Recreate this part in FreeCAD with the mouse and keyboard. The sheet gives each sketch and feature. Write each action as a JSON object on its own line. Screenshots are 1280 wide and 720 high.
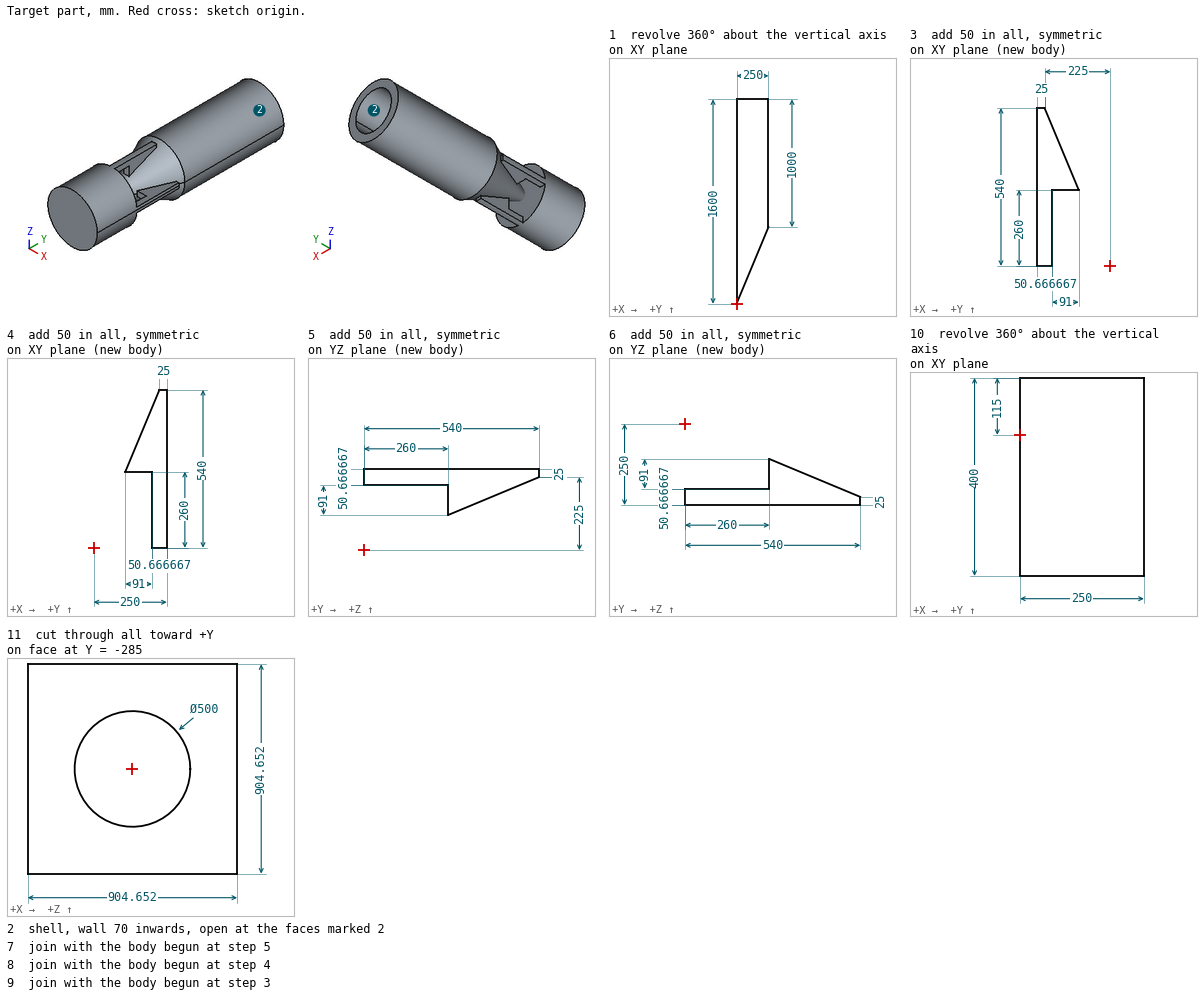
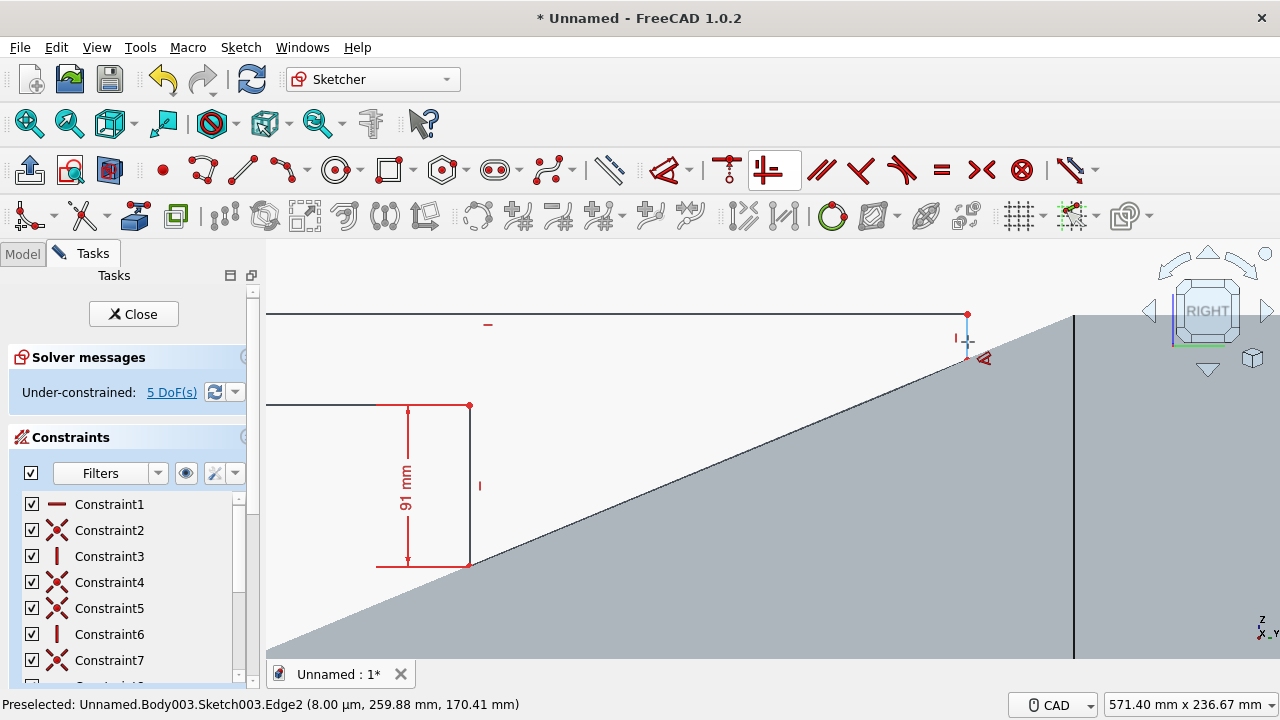
{"action": "left_click", "coordinate": [967, 342]}
{"action": "left_click", "coordinate": [1001, 337]}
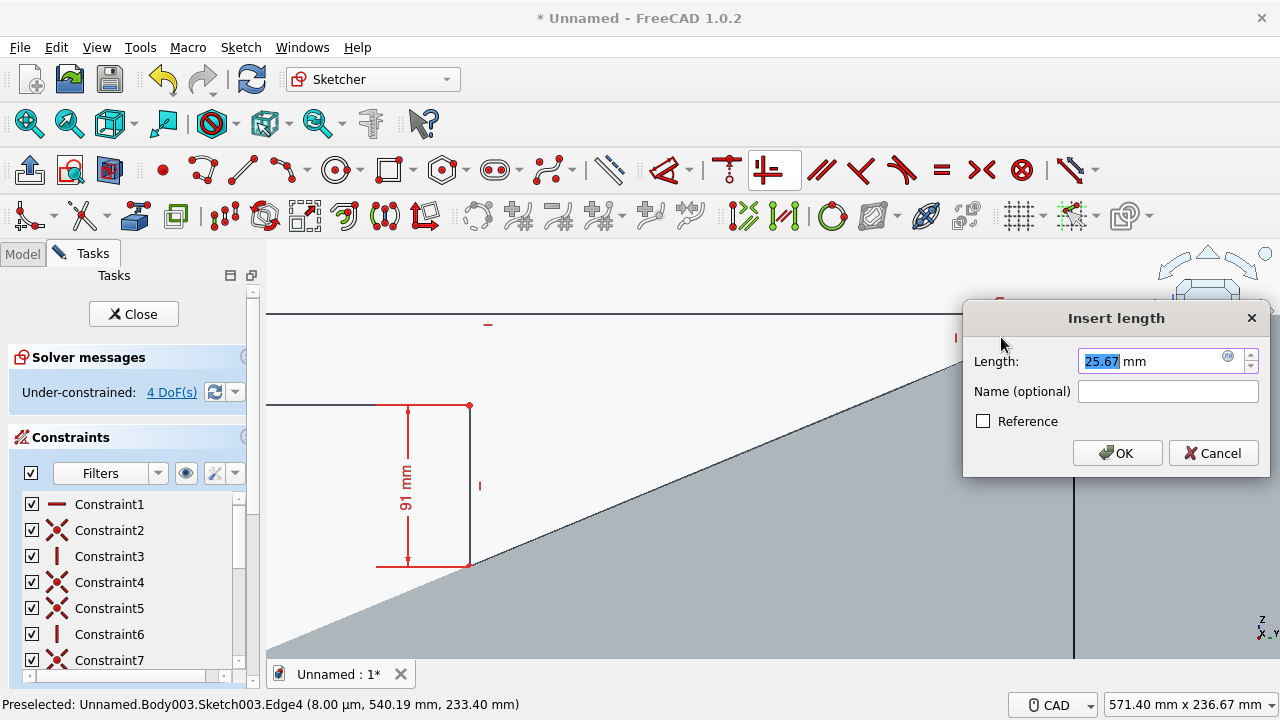
{"action": "type", "text": "25"}
{"action": "key", "text": "Return"}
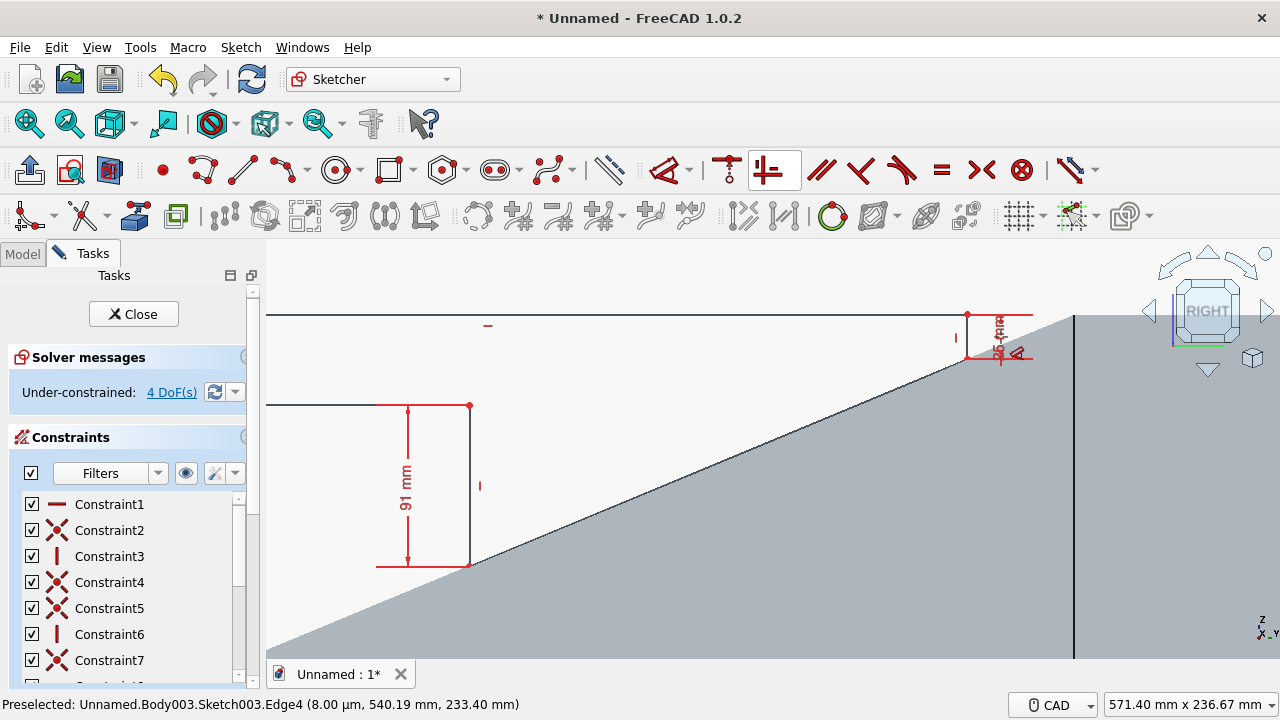
{"action": "left_click", "coordinate": [332, 405]}
{"action": "left_click", "coordinate": [382, 371]}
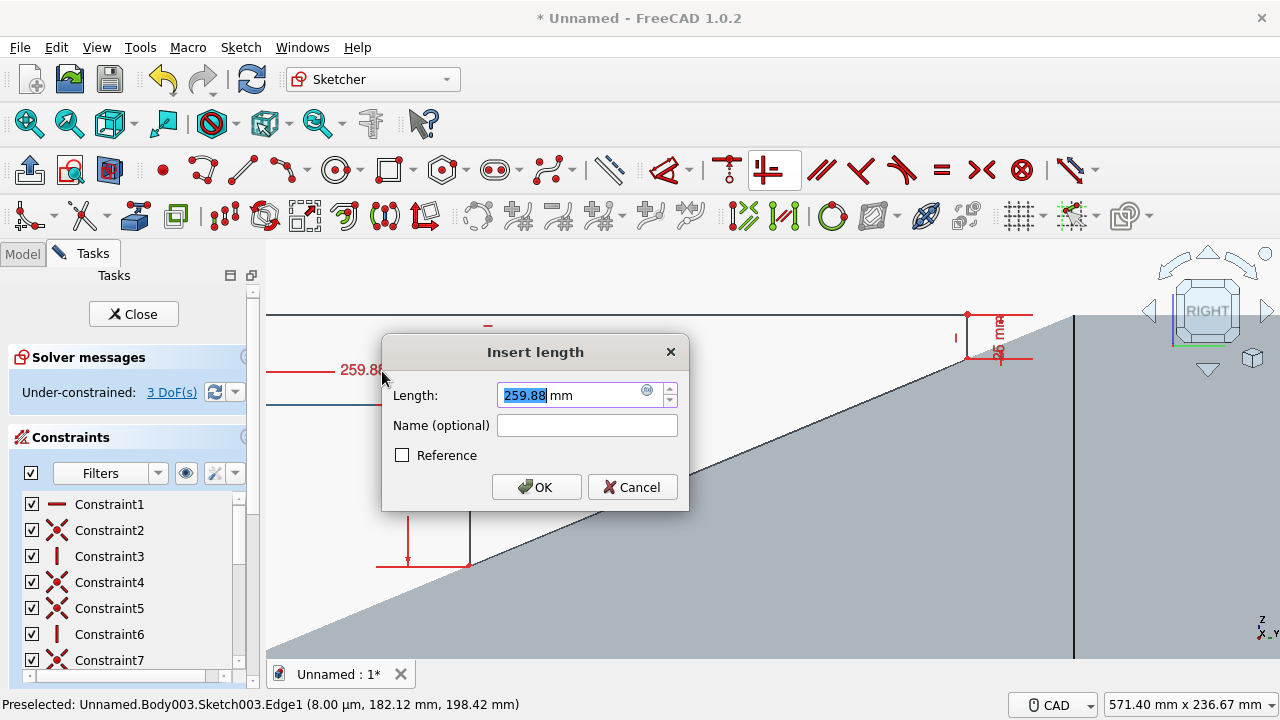
{"action": "type", "text": "260"}
{"action": "key", "text": "Return"}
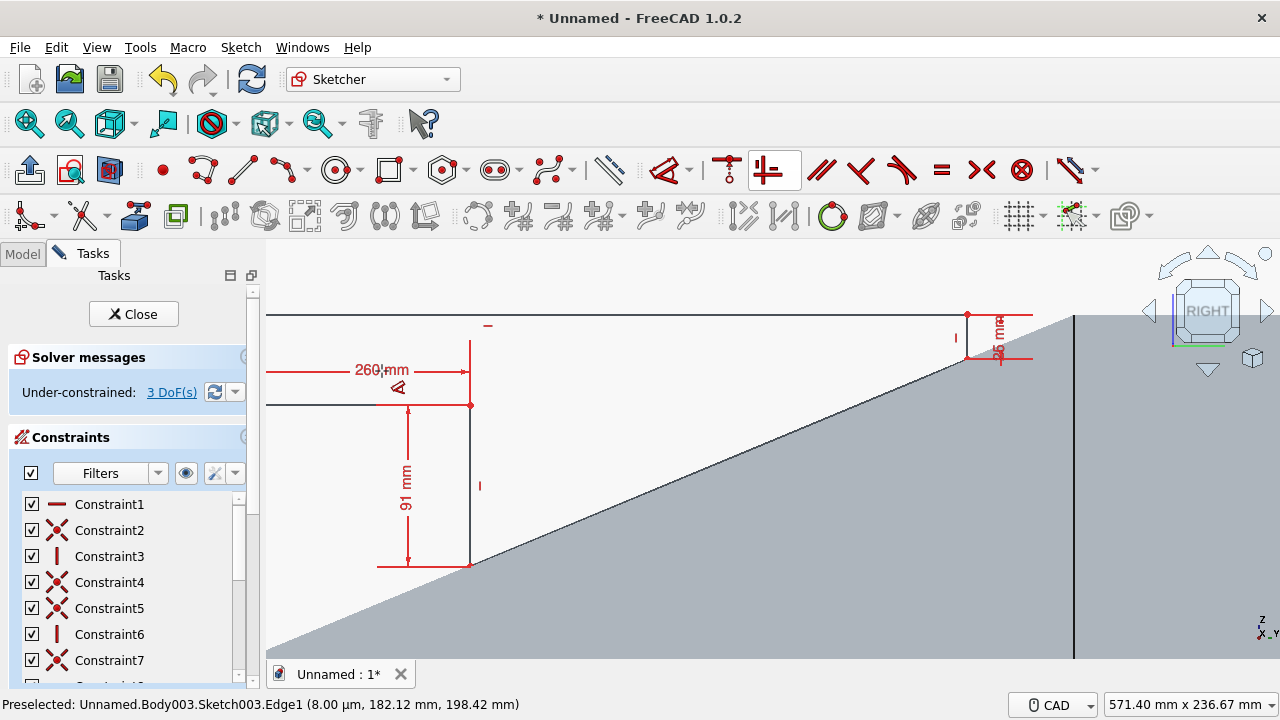
{"action": "left_click", "coordinate": [680, 315]}
{"action": "left_click", "coordinate": [631, 281]}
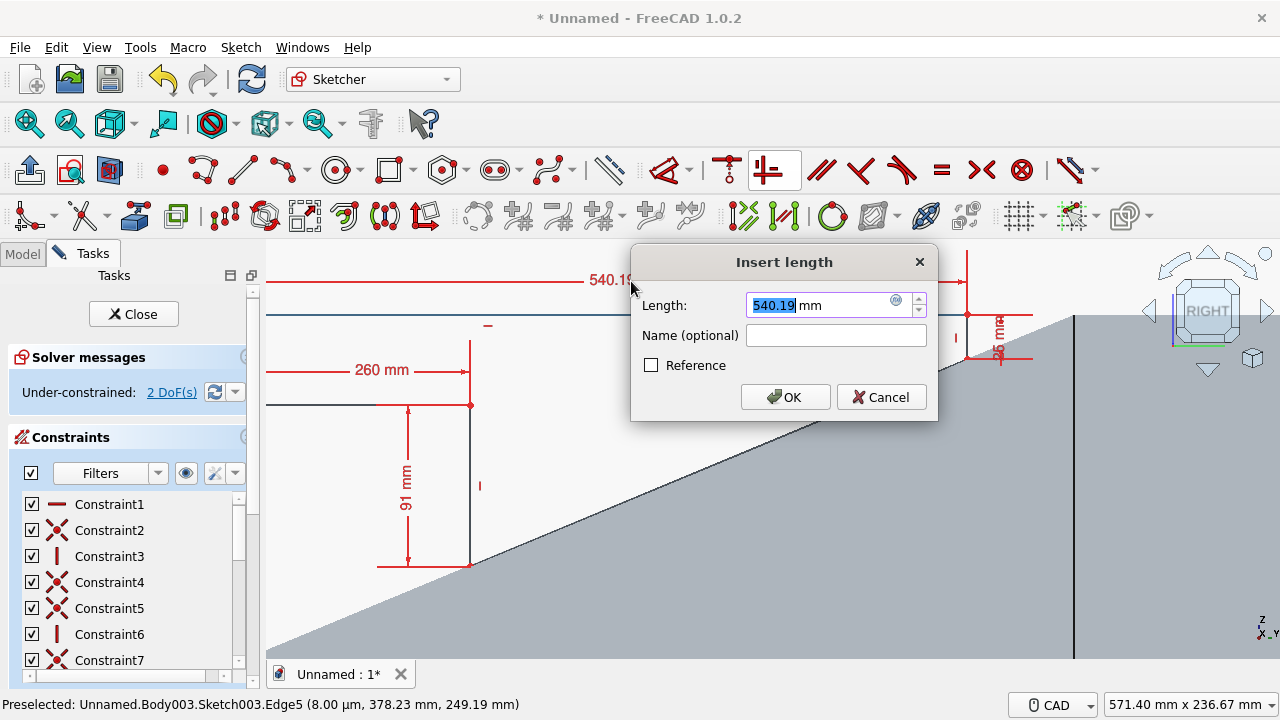
{"action": "type", "text": "540"}
{"action": "key", "text": "Return"}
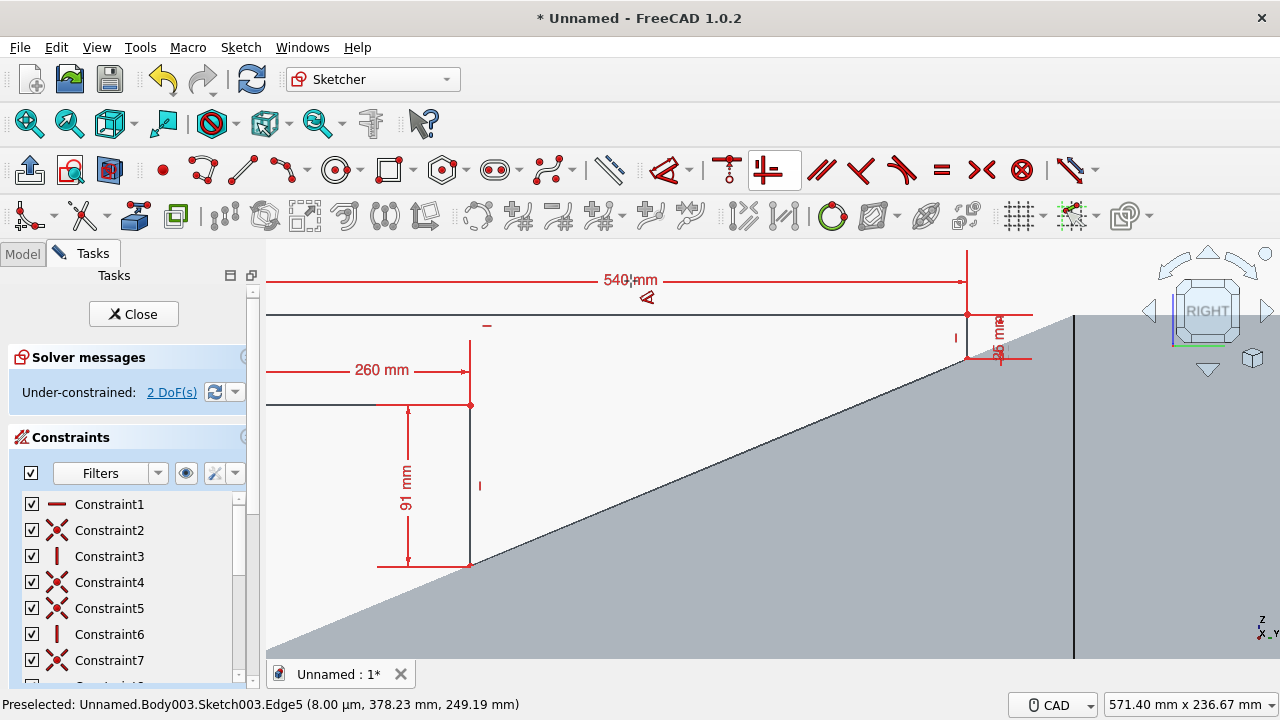
{"action": "left_click", "coordinate": [967, 359]}
{"action": "left_click", "coordinate": [1001, 495]}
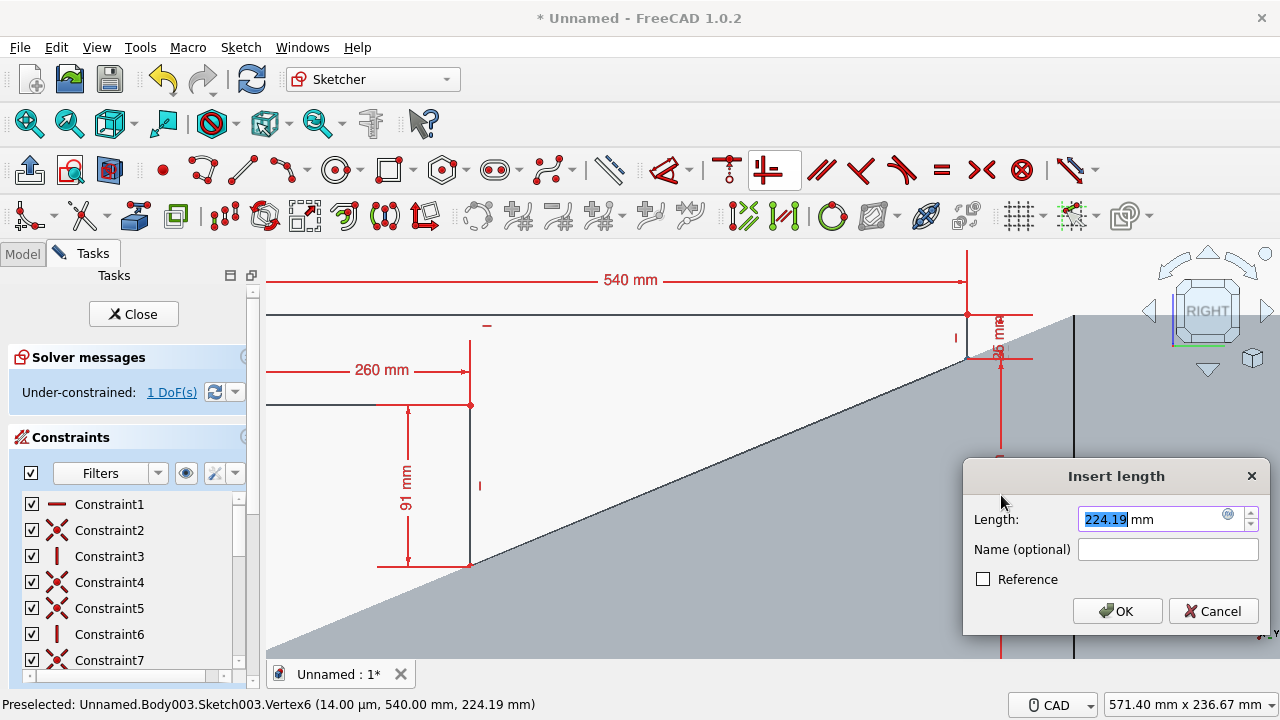
{"action": "type", "text": "225"}
{"action": "key", "text": "Return"}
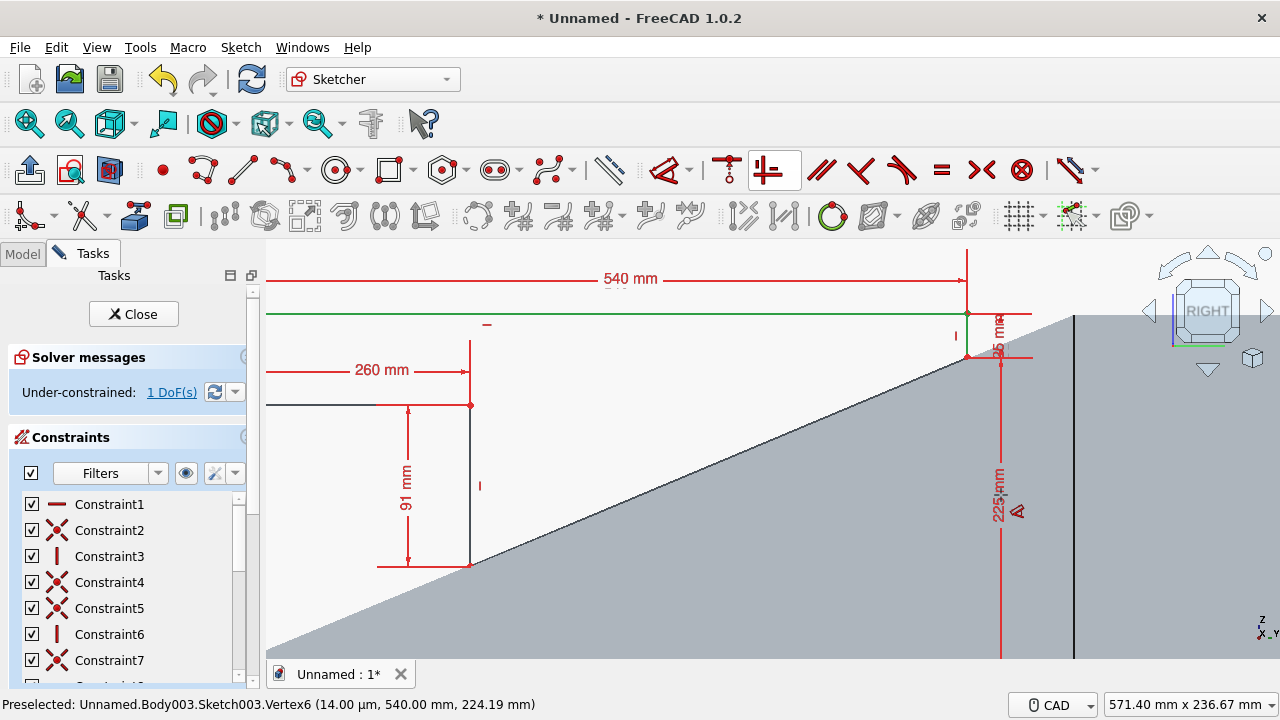
{"action": "scroll", "coordinate": [968, 344], "scroll_direction": "down", "scroll_amount": 3}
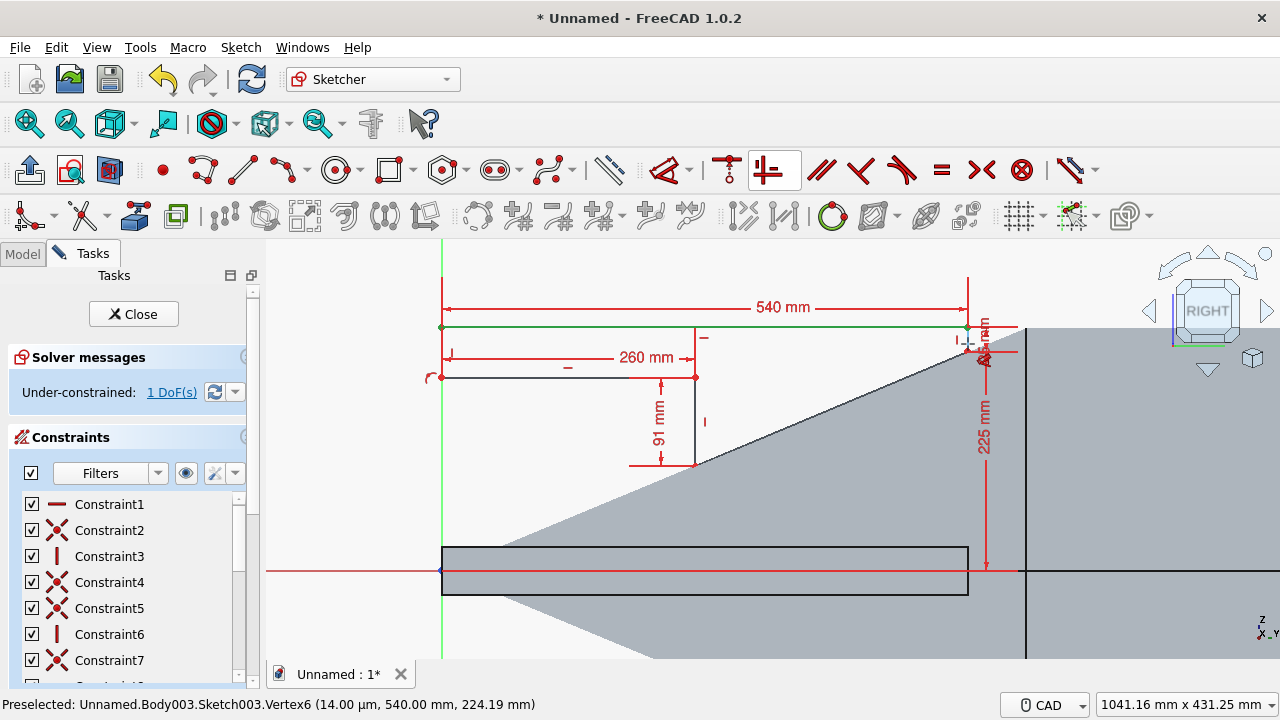
{"action": "left_click", "coordinate": [442, 342]}
{"action": "left_click", "coordinate": [408, 353]}